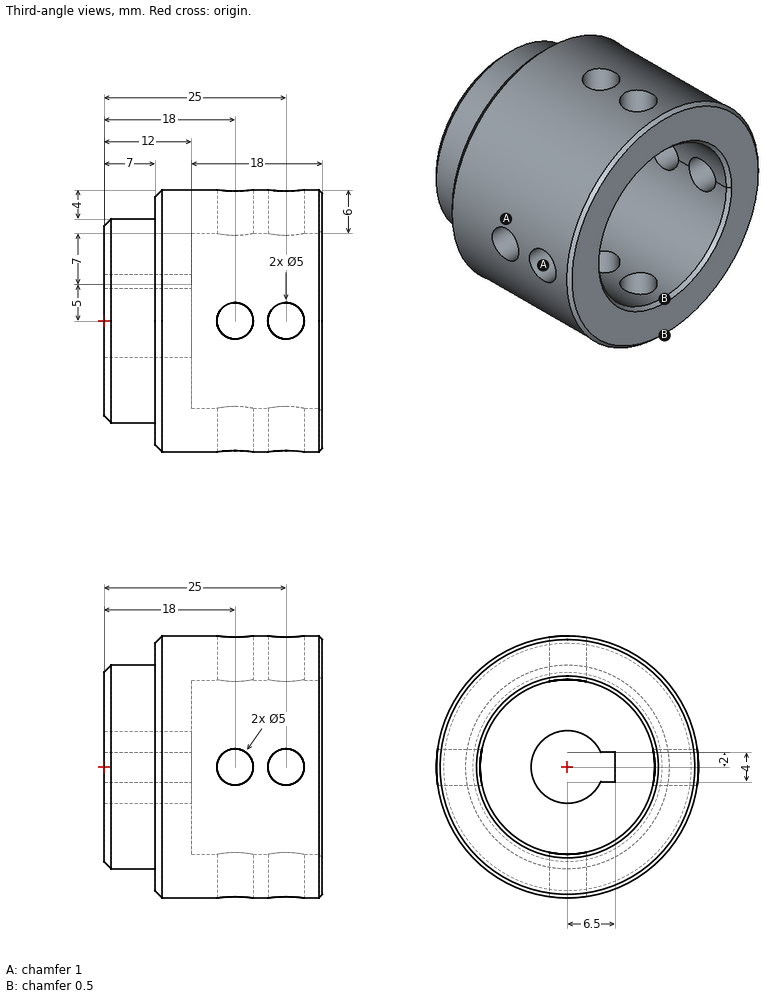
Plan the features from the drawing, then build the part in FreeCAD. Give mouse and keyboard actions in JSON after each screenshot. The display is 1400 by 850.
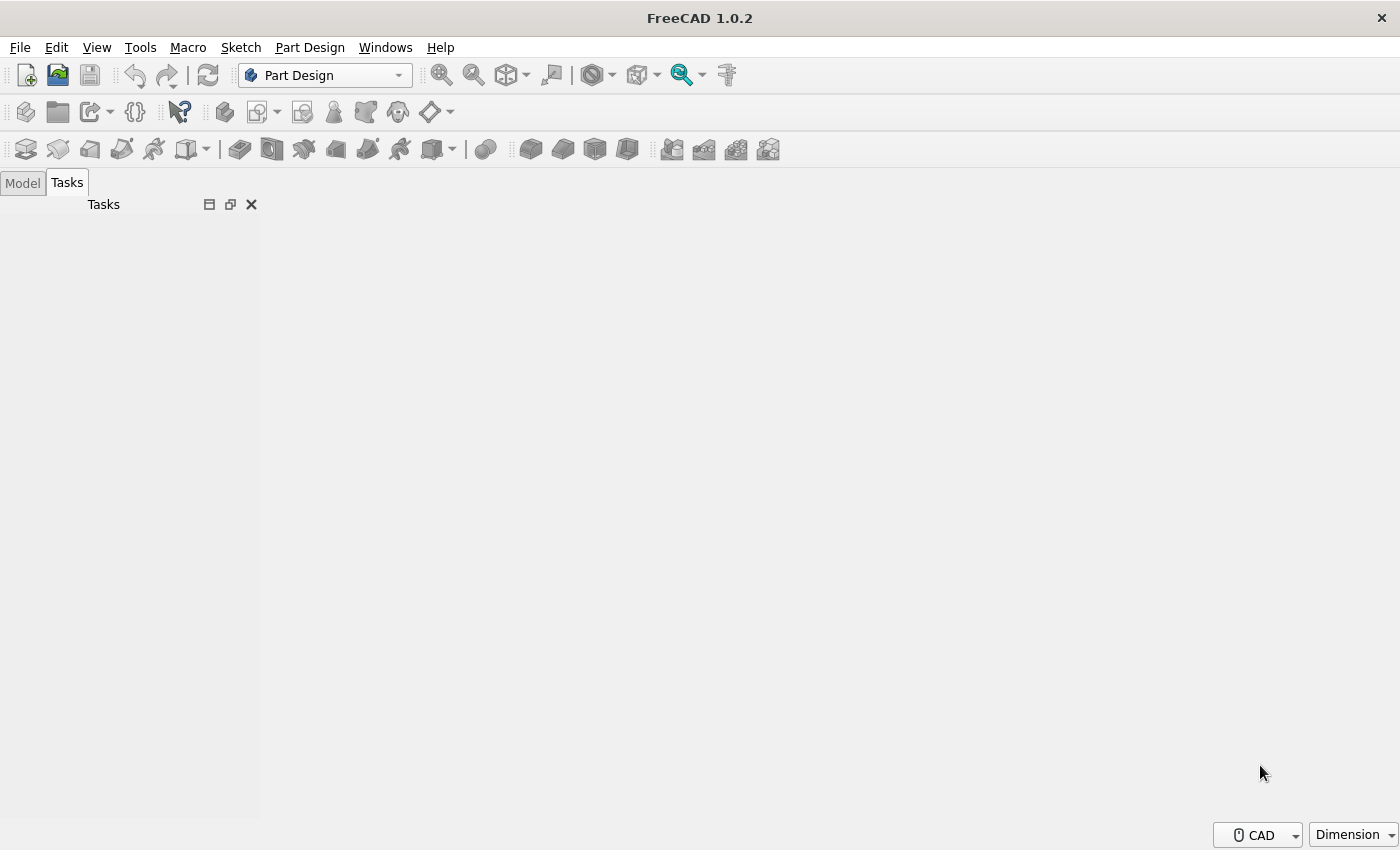
{"action": "left_click", "coordinate": [26, 76]}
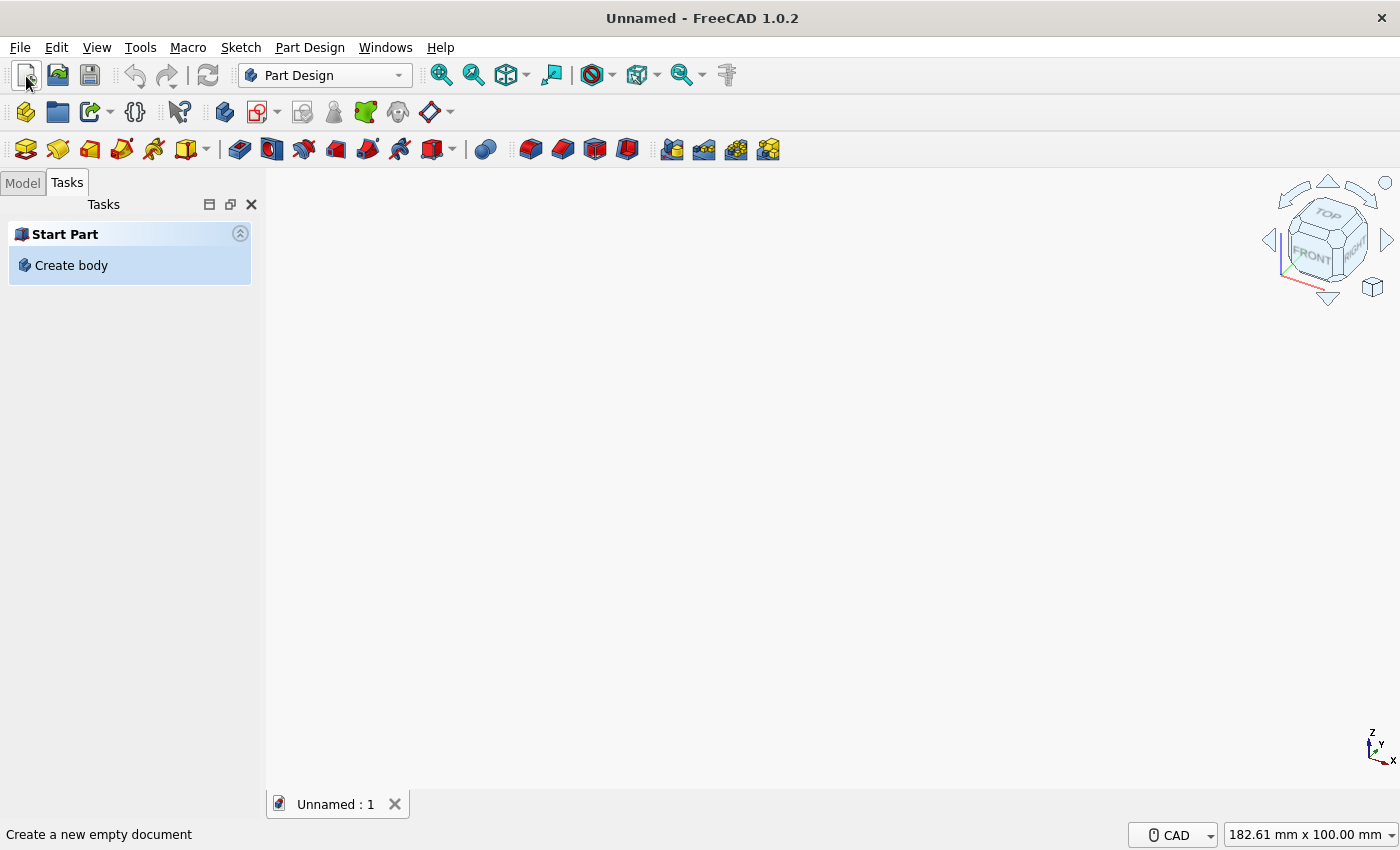
{"action": "left_click", "coordinate": [258, 112]}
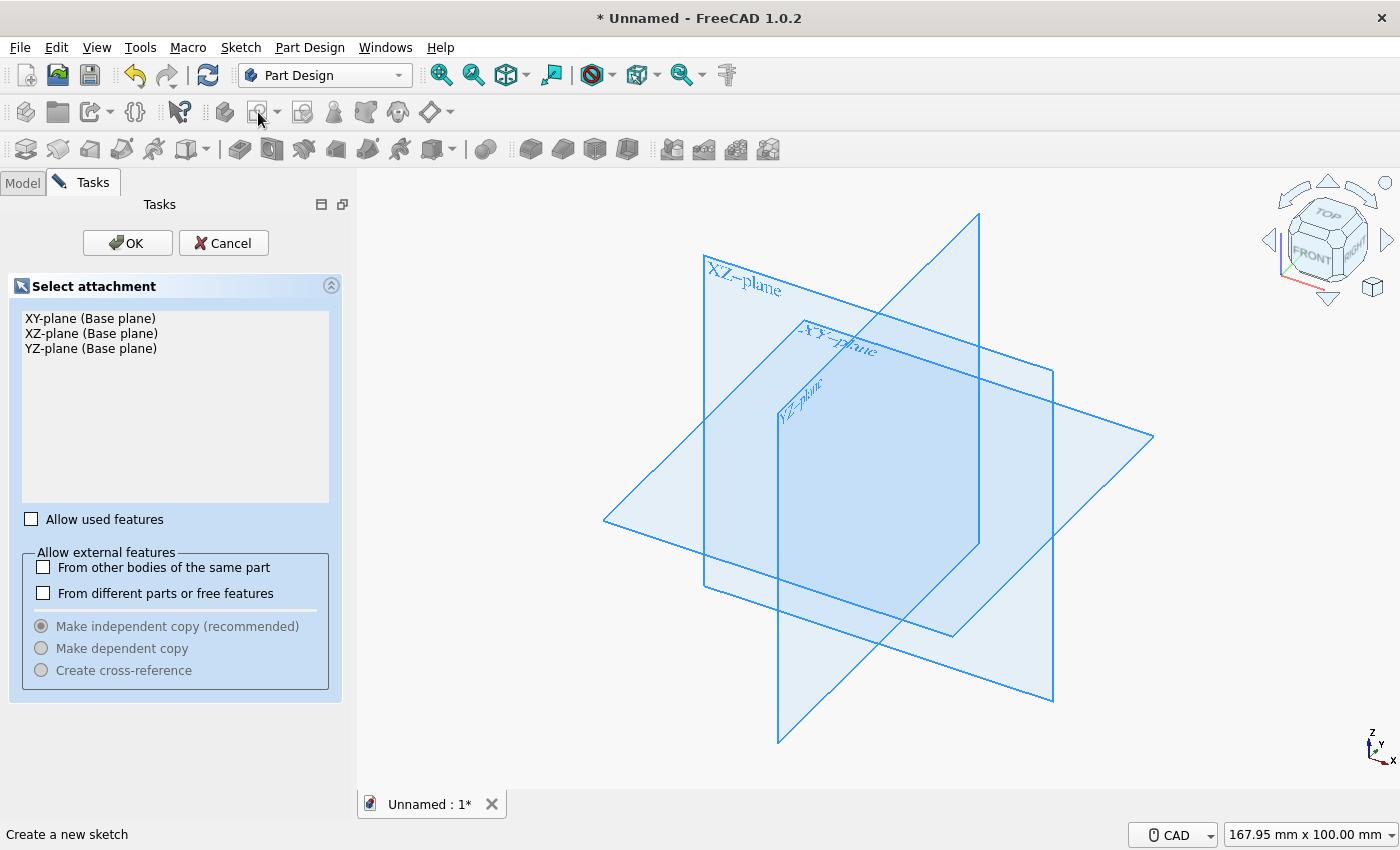
{"action": "left_click", "coordinate": [82, 318]}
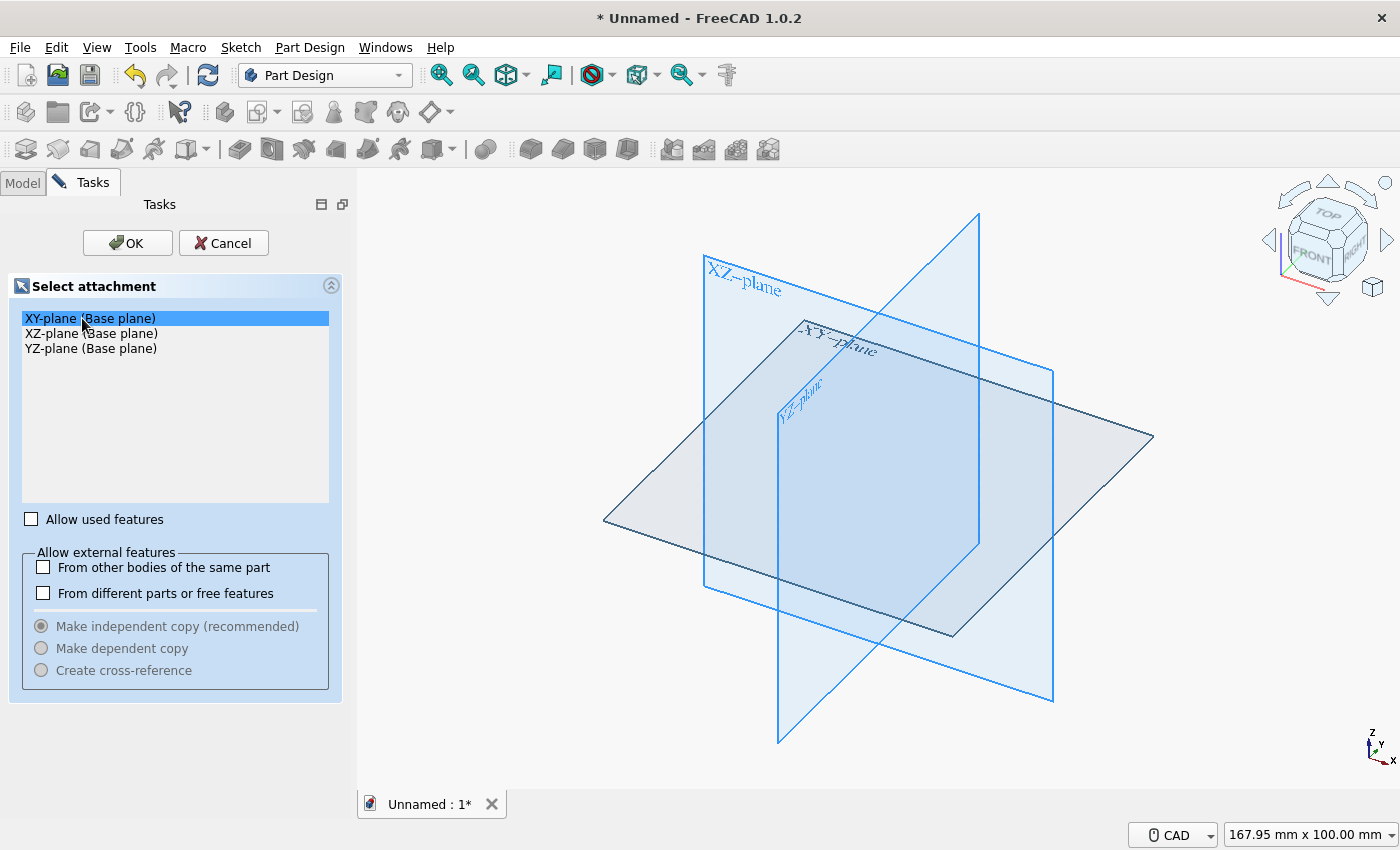
{"action": "left_click", "coordinate": [128, 243]}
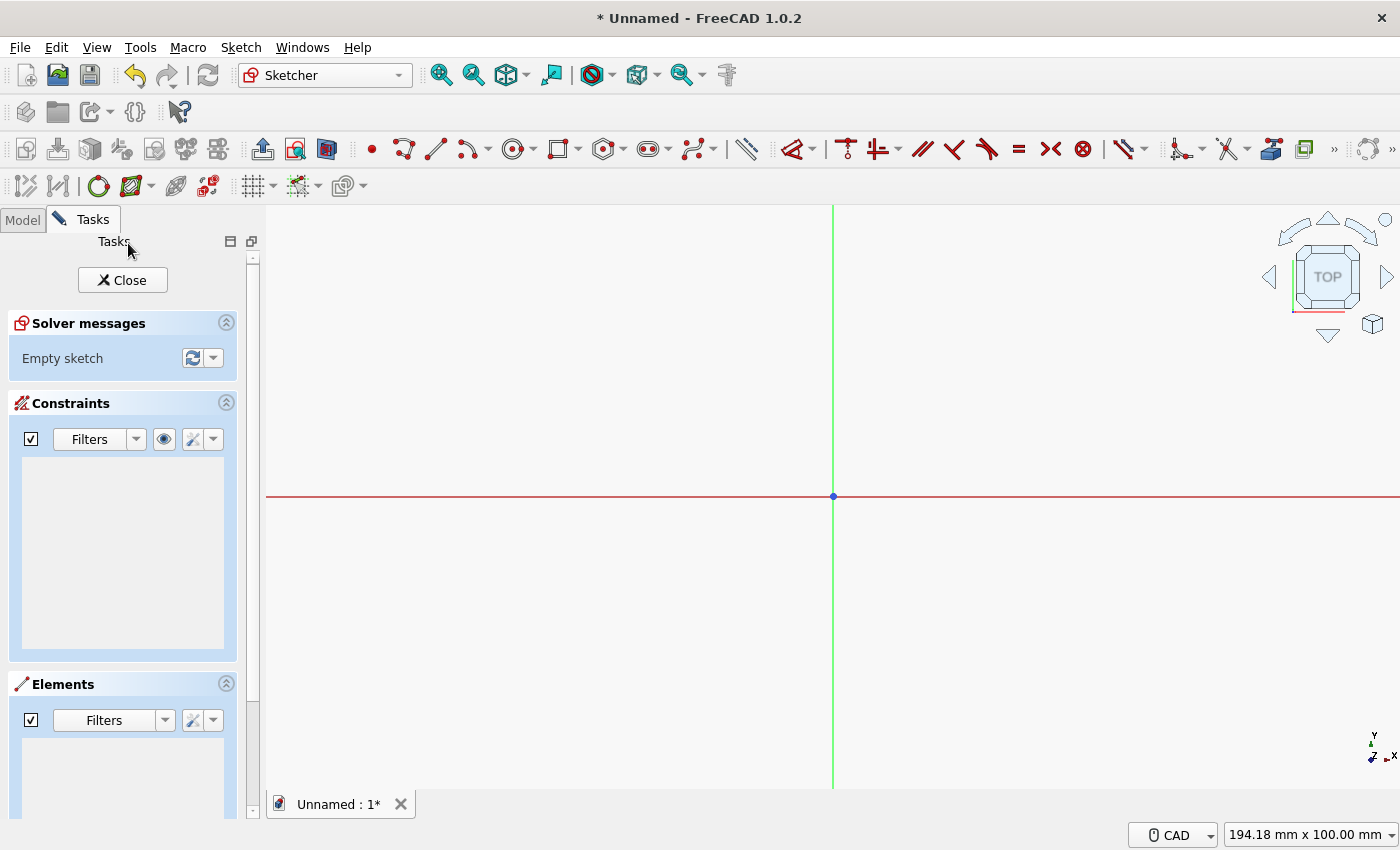
{"action": "scroll", "coordinate": [988, 422], "scroll_direction": "up", "scroll_amount": 6}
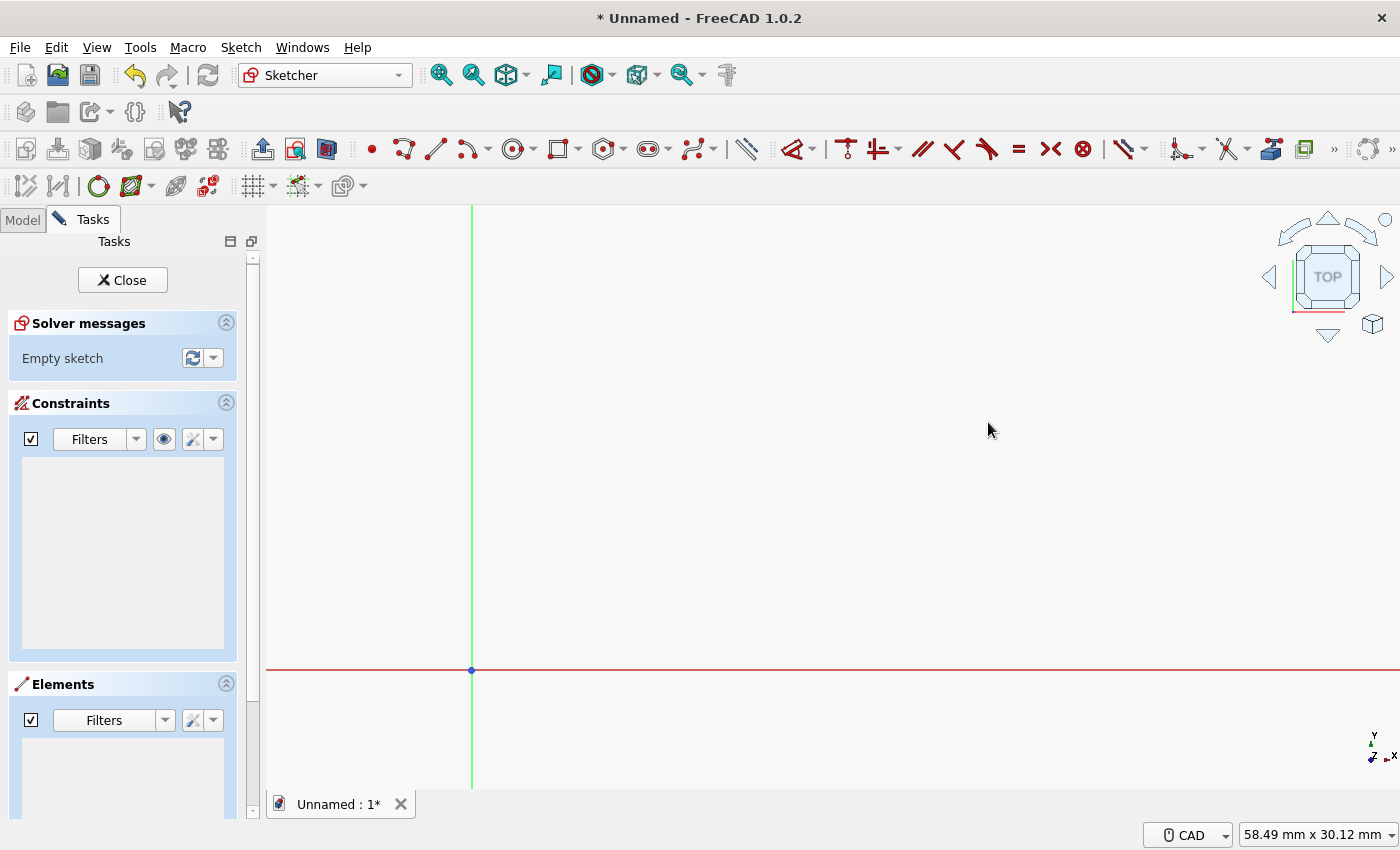
{"action": "left_click", "coordinate": [404, 150]}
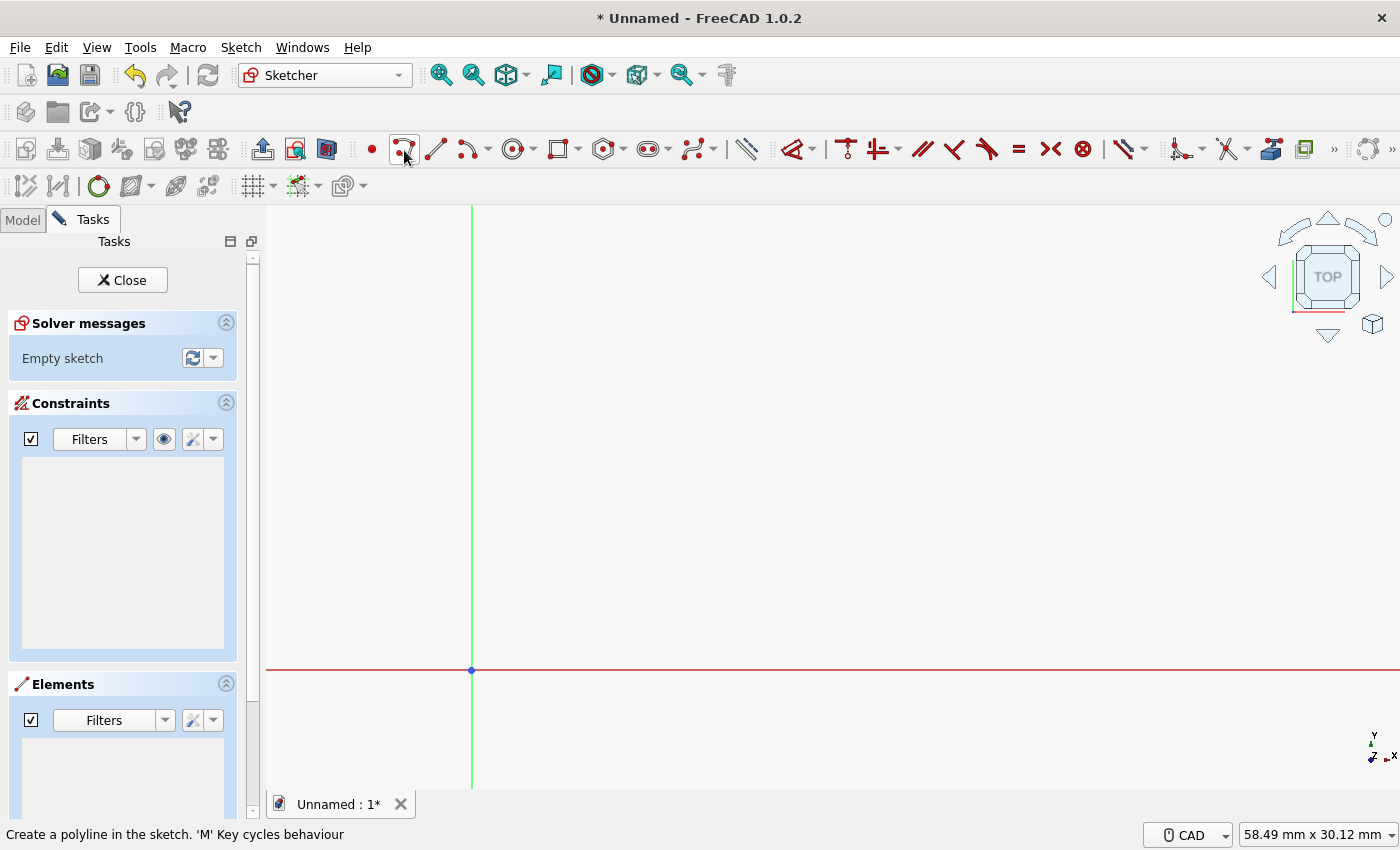
{"action": "left_click", "coordinate": [472, 573]}
{"action": "left_click", "coordinate": [705, 573]}
{"action": "left_click", "coordinate": [705, 437]}
{"action": "left_click", "coordinate": [1054, 437]}
{"action": "left_click", "coordinate": [1054, 321]}
{"action": "left_click", "coordinate": [608, 321]}
{"action": "left_click", "coordinate": [608, 399]}
{"action": "left_click", "coordinate": [481, 399]}
{"action": "left_click", "coordinate": [472, 574]}
{"action": "key", "text": "Escape"}
{"action": "key", "text": "Escape"}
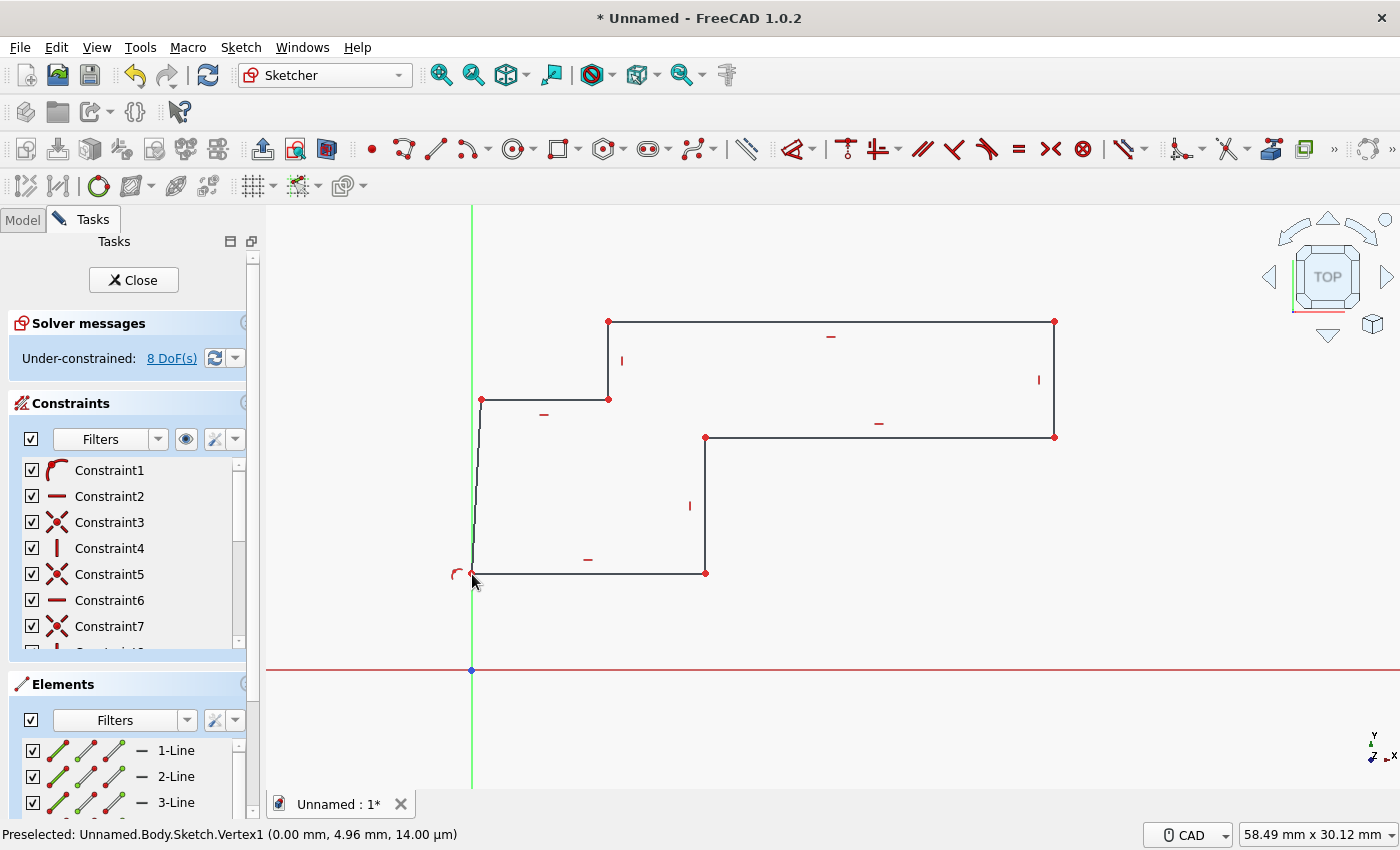
{"action": "left_click", "coordinate": [475, 522]}